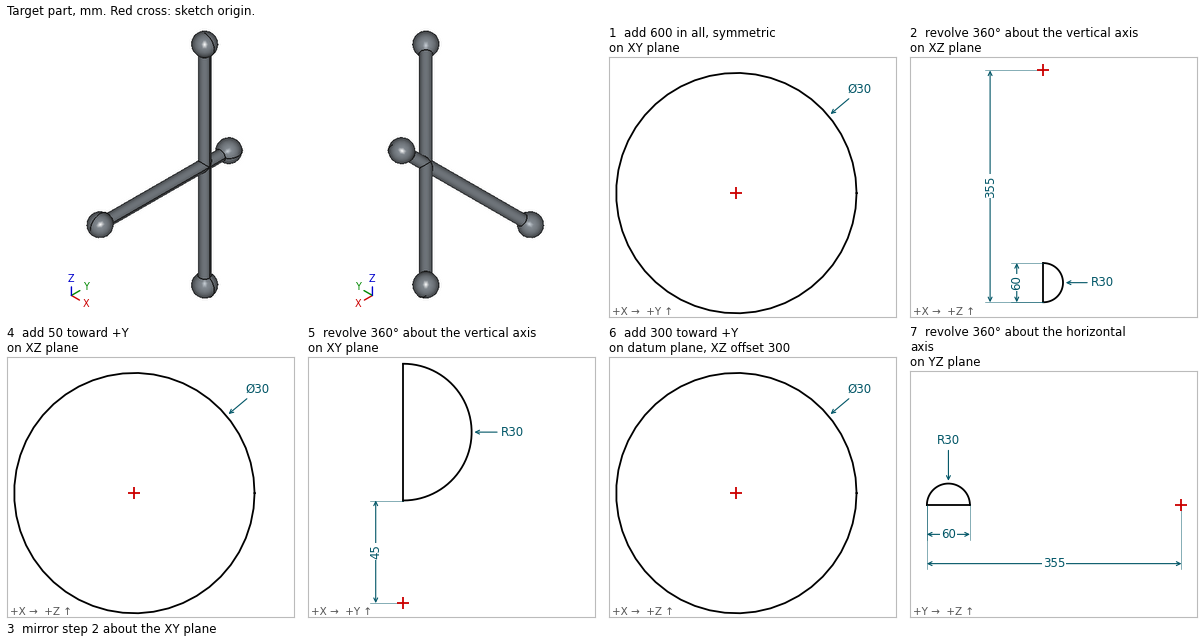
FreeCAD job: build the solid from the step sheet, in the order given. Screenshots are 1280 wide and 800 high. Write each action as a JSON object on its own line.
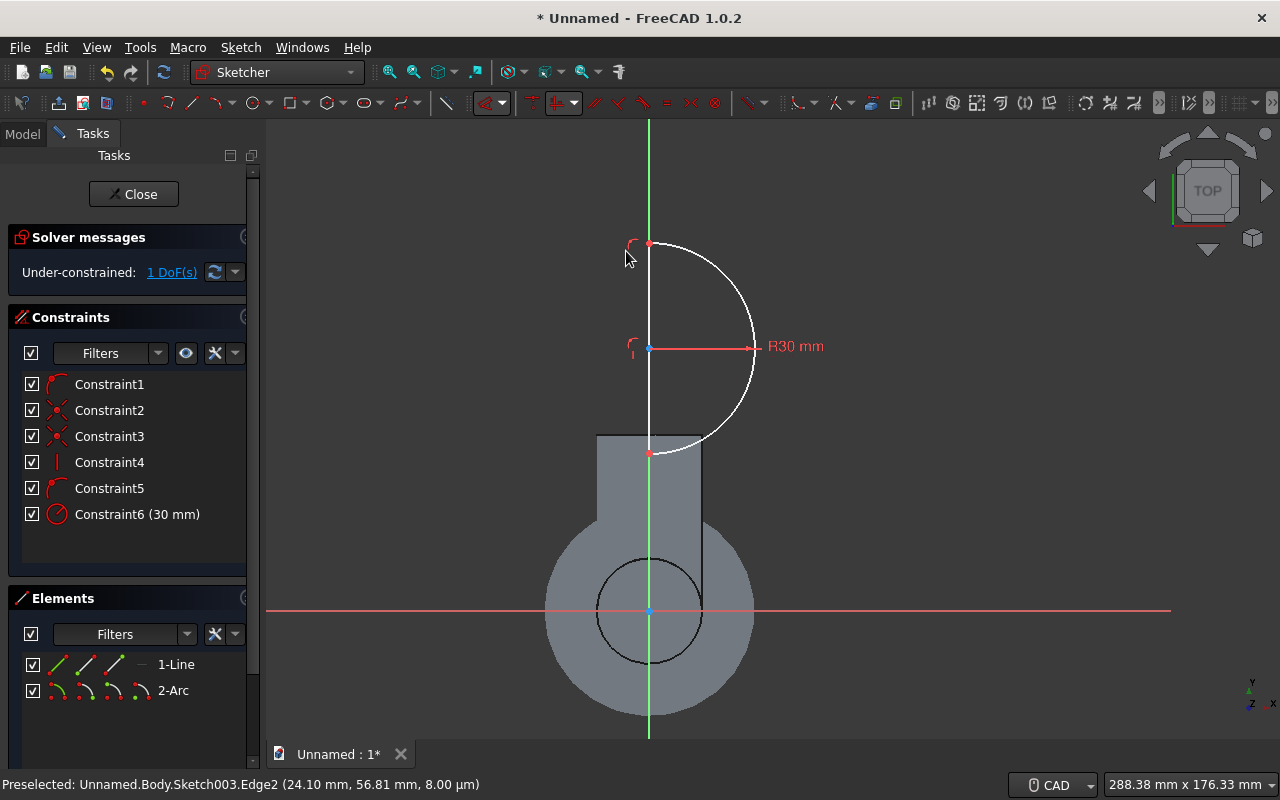
{"action": "left_click", "coordinate": [649, 454]}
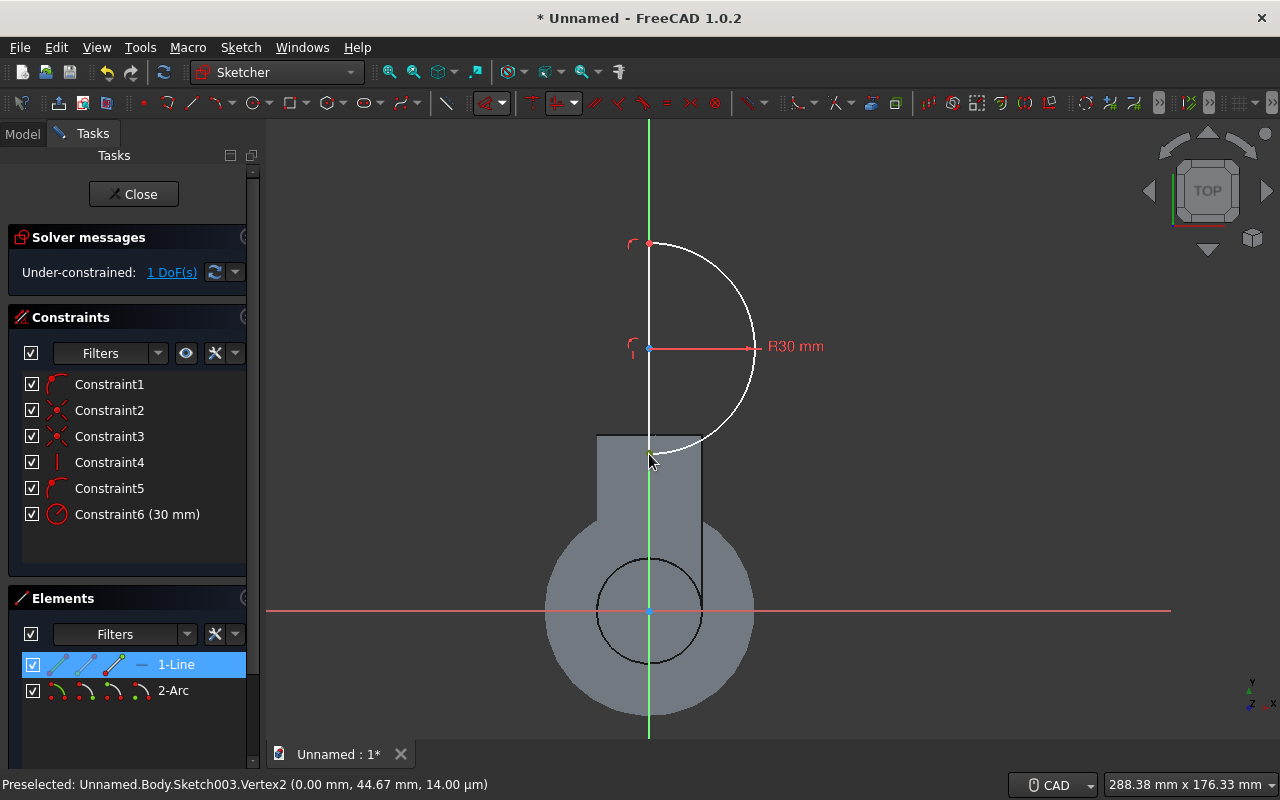
{"action": "key", "text": "i"}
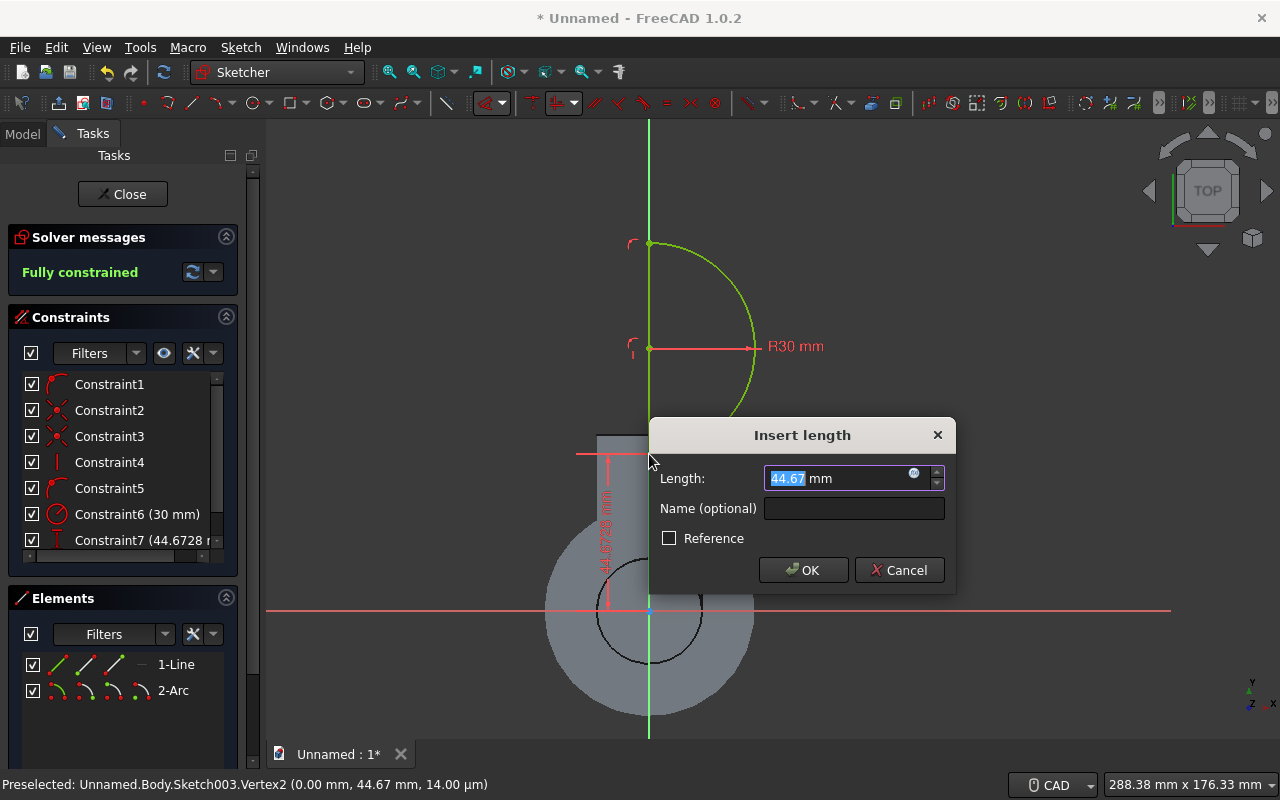
{"action": "type", "text": "45"}
{"action": "key", "text": "Return"}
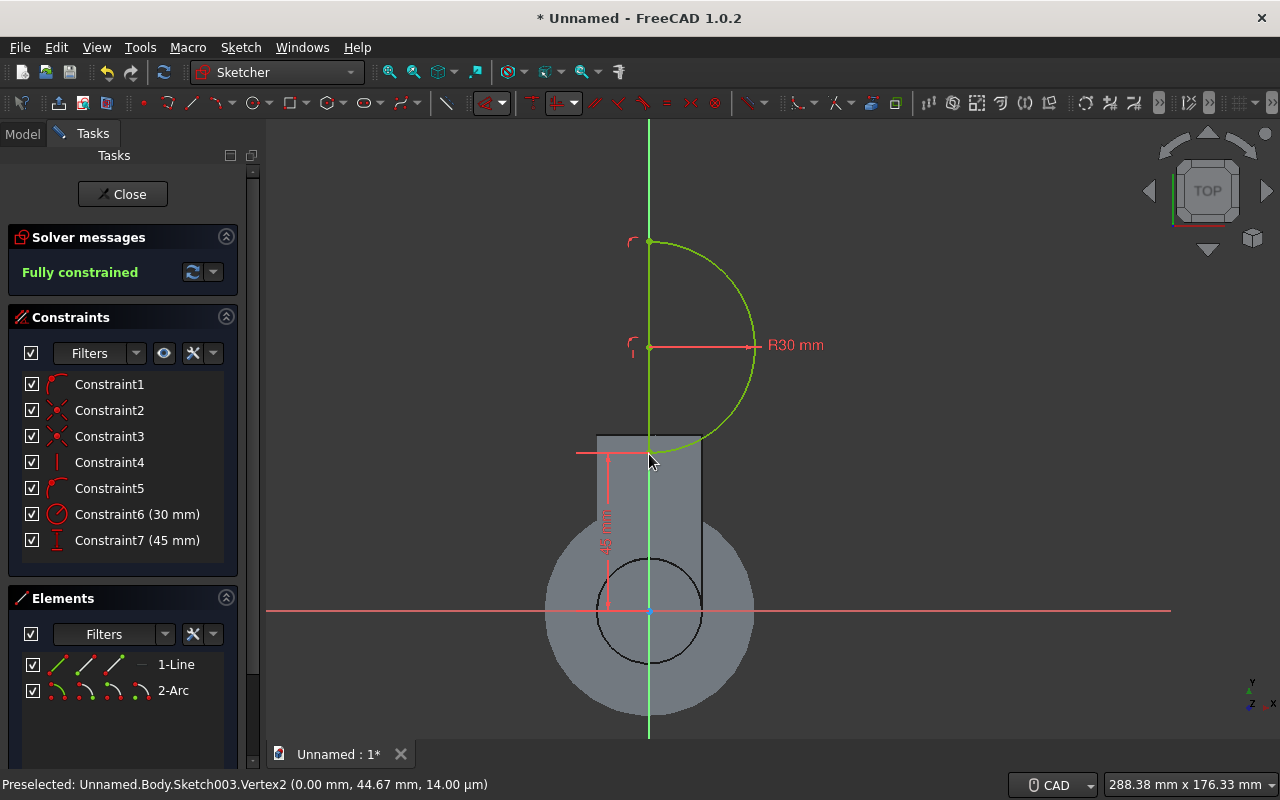
{"action": "left_click", "coordinate": [123, 194]}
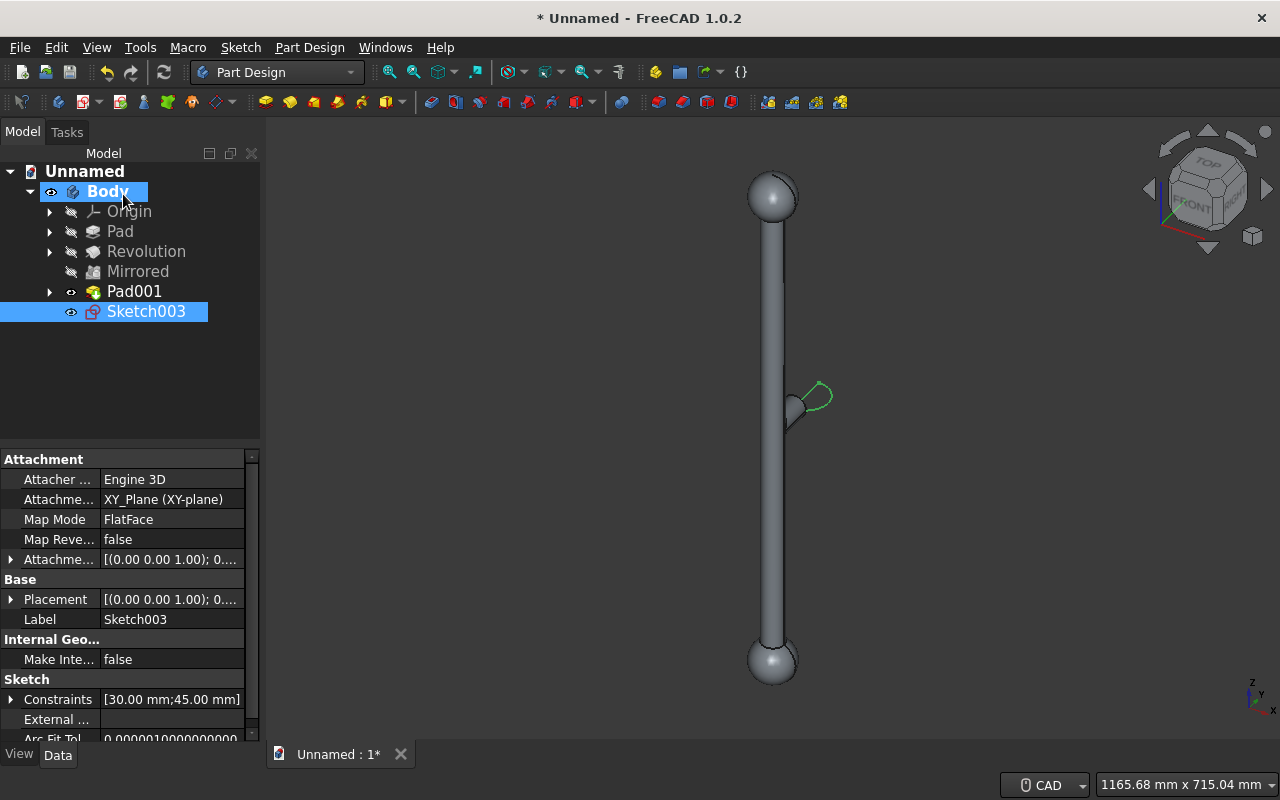
{"action": "left_click", "coordinate": [290, 102]}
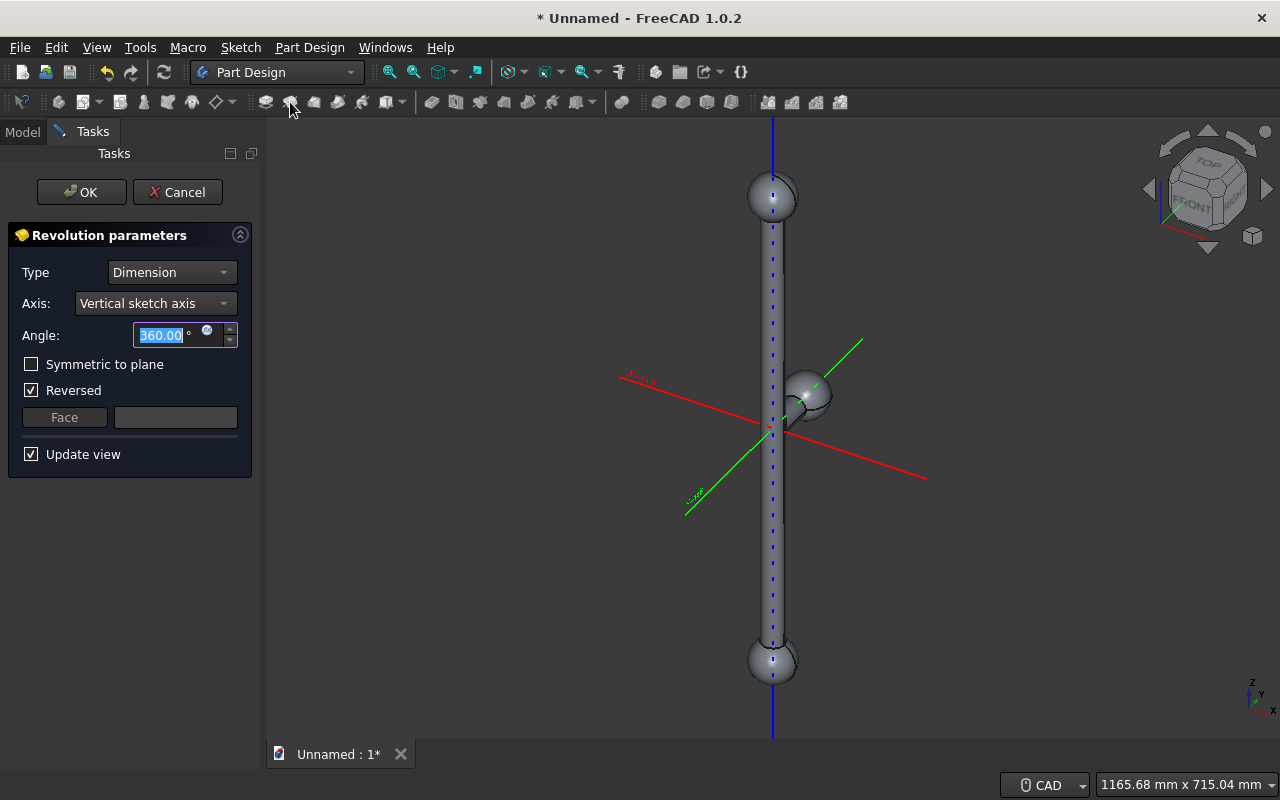
{"action": "left_click", "coordinate": [82, 192]}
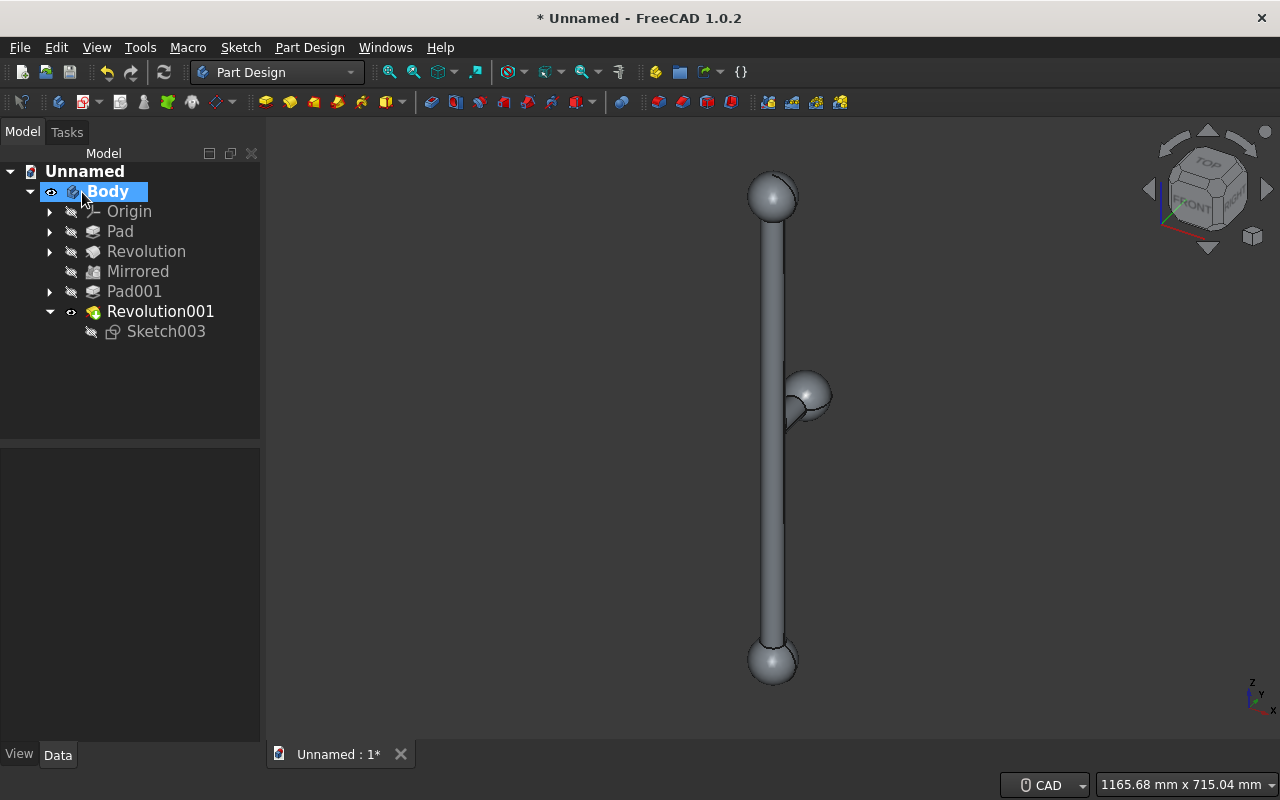
{"action": "left_click", "coordinate": [50, 212]}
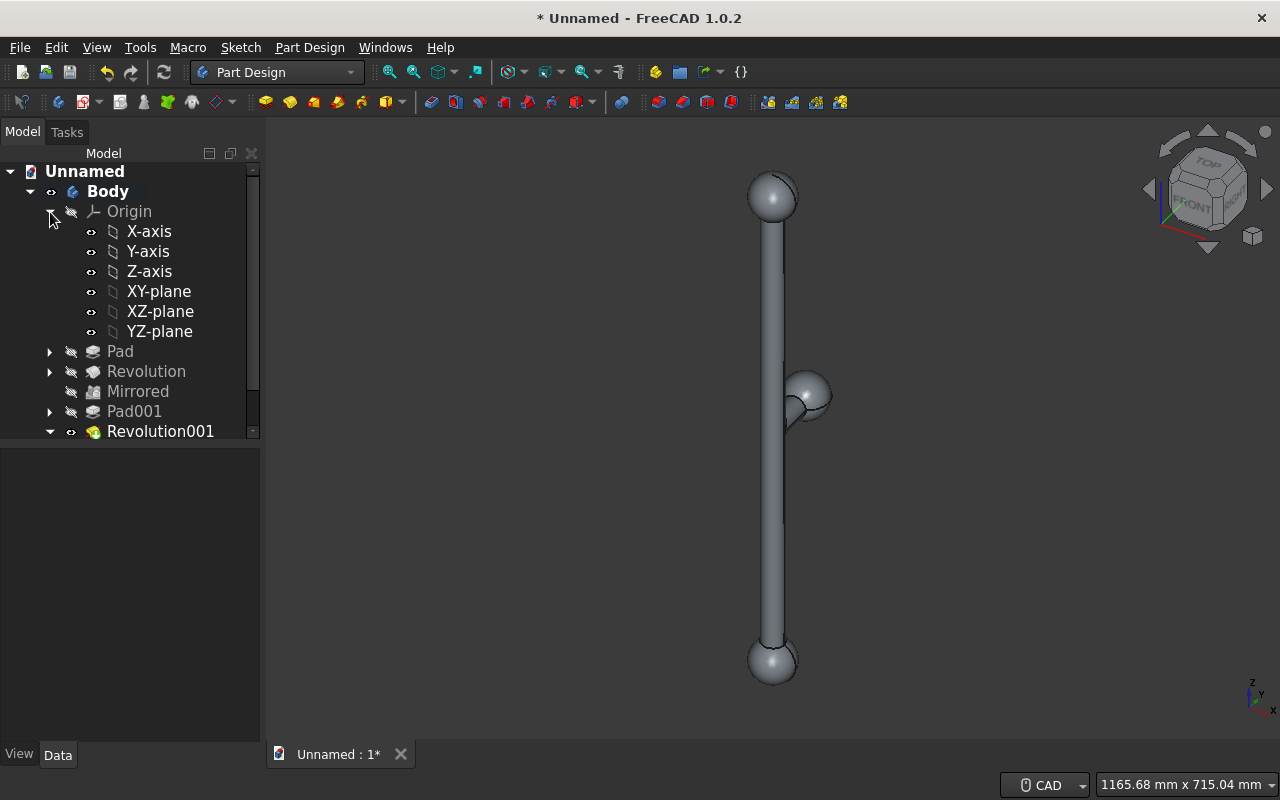
{"action": "left_click", "coordinate": [136, 312]}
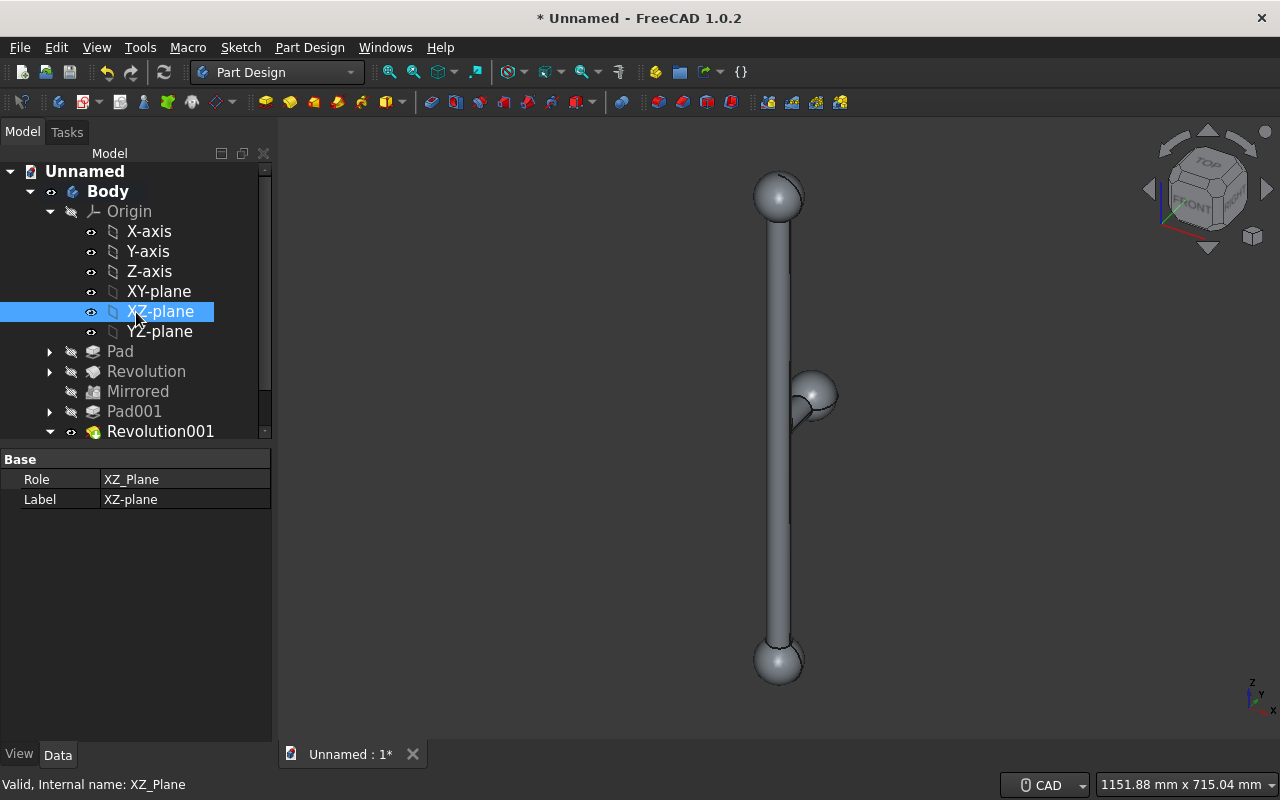
{"action": "left_click", "coordinate": [216, 102]}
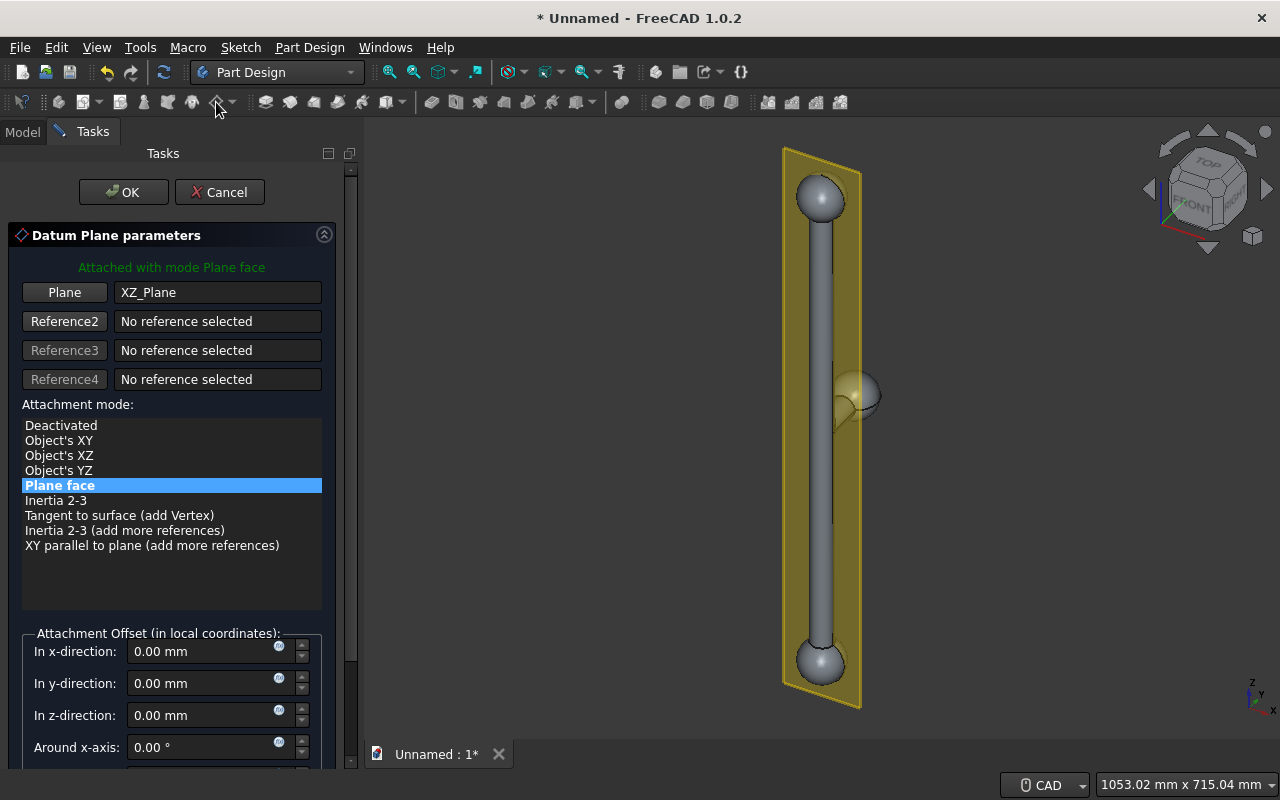
{"action": "triple_click", "coordinate": [210, 715]}